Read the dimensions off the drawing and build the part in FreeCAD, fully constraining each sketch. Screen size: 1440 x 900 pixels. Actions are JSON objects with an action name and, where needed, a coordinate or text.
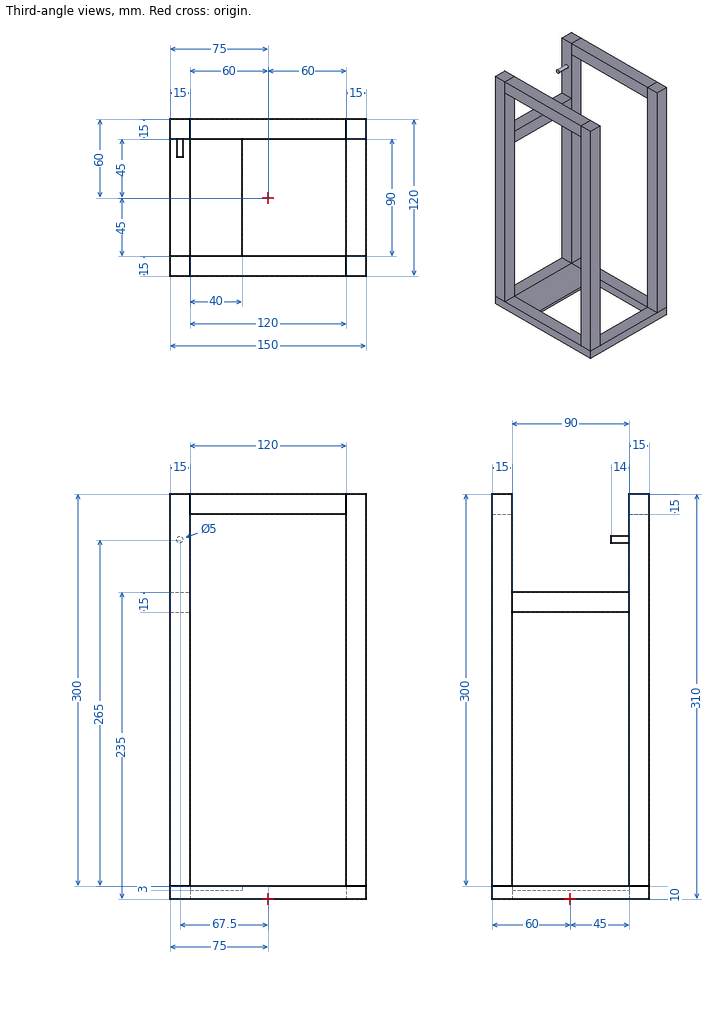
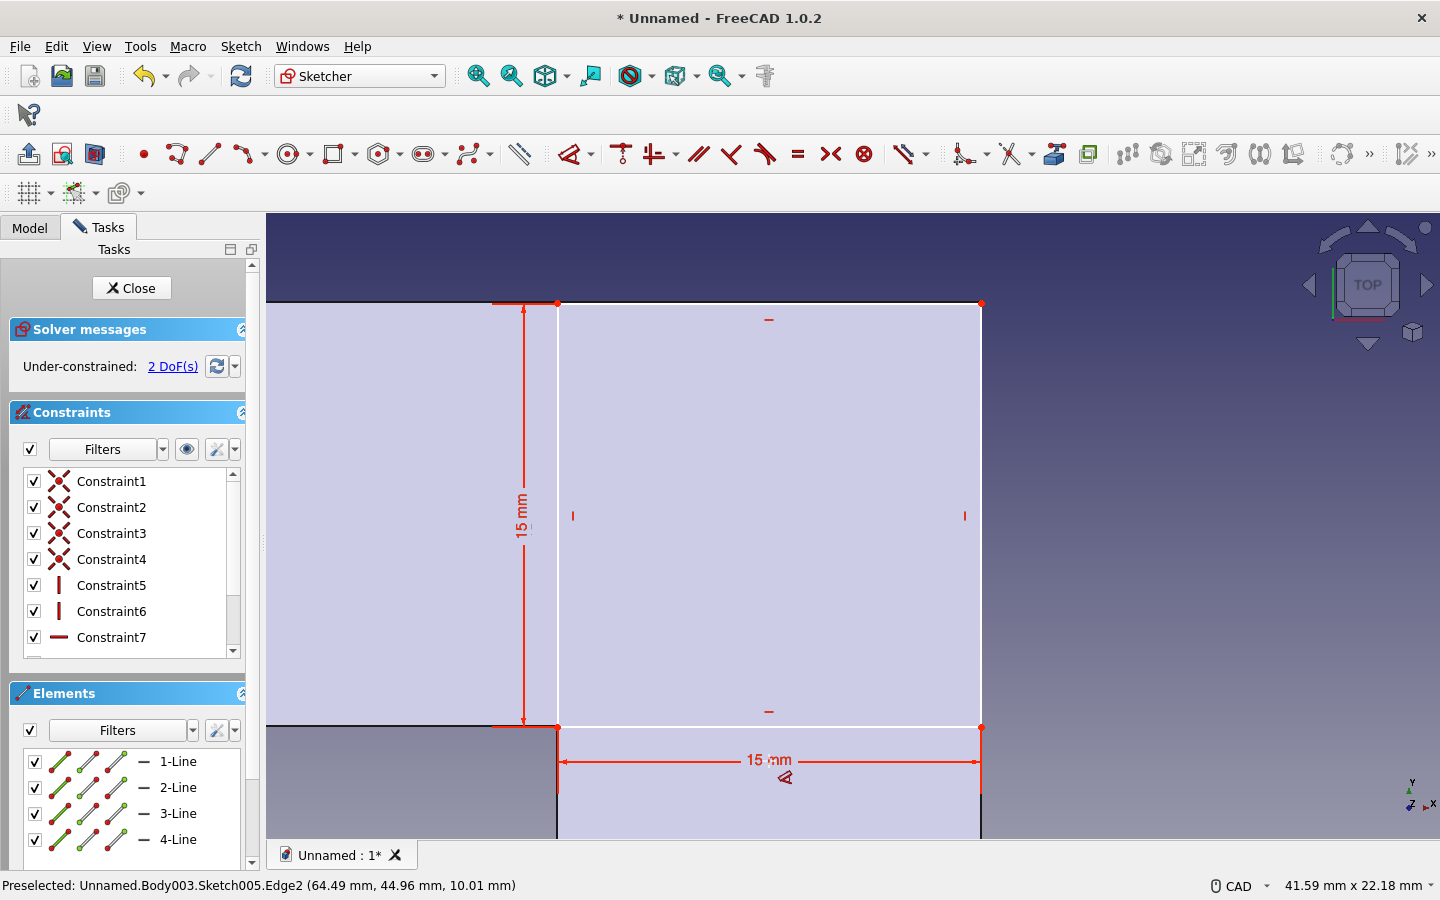
{"action": "left_click", "coordinate": [558, 304]}
{"action": "left_click", "coordinate": [426, 270]}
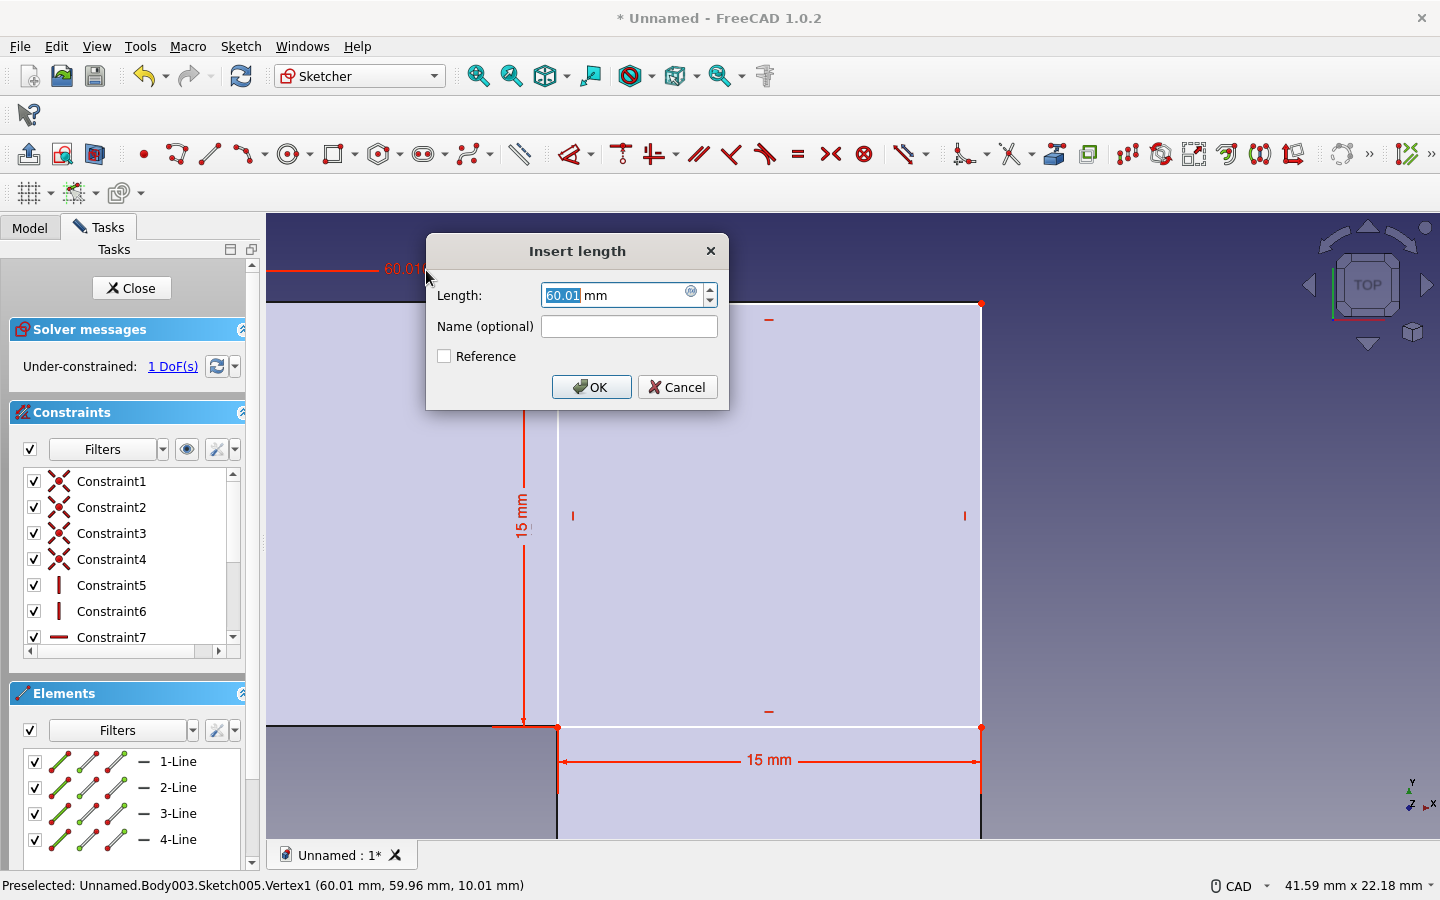
{"action": "type", "text": "60"}
{"action": "key", "text": "Return"}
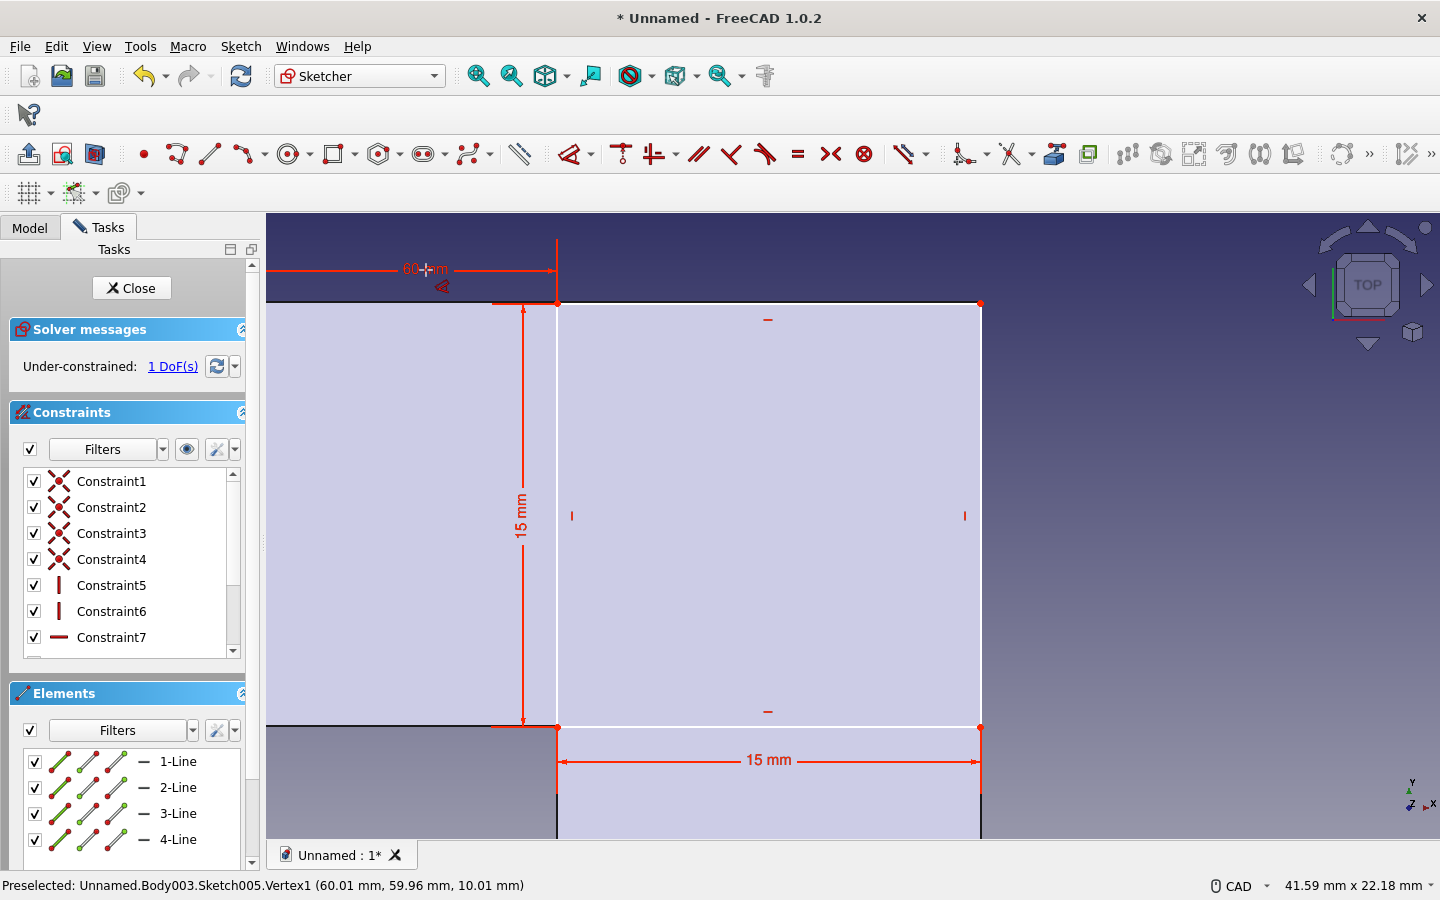
{"action": "left_click", "coordinate": [557, 304]}
{"action": "left_click", "coordinate": [591, 557]}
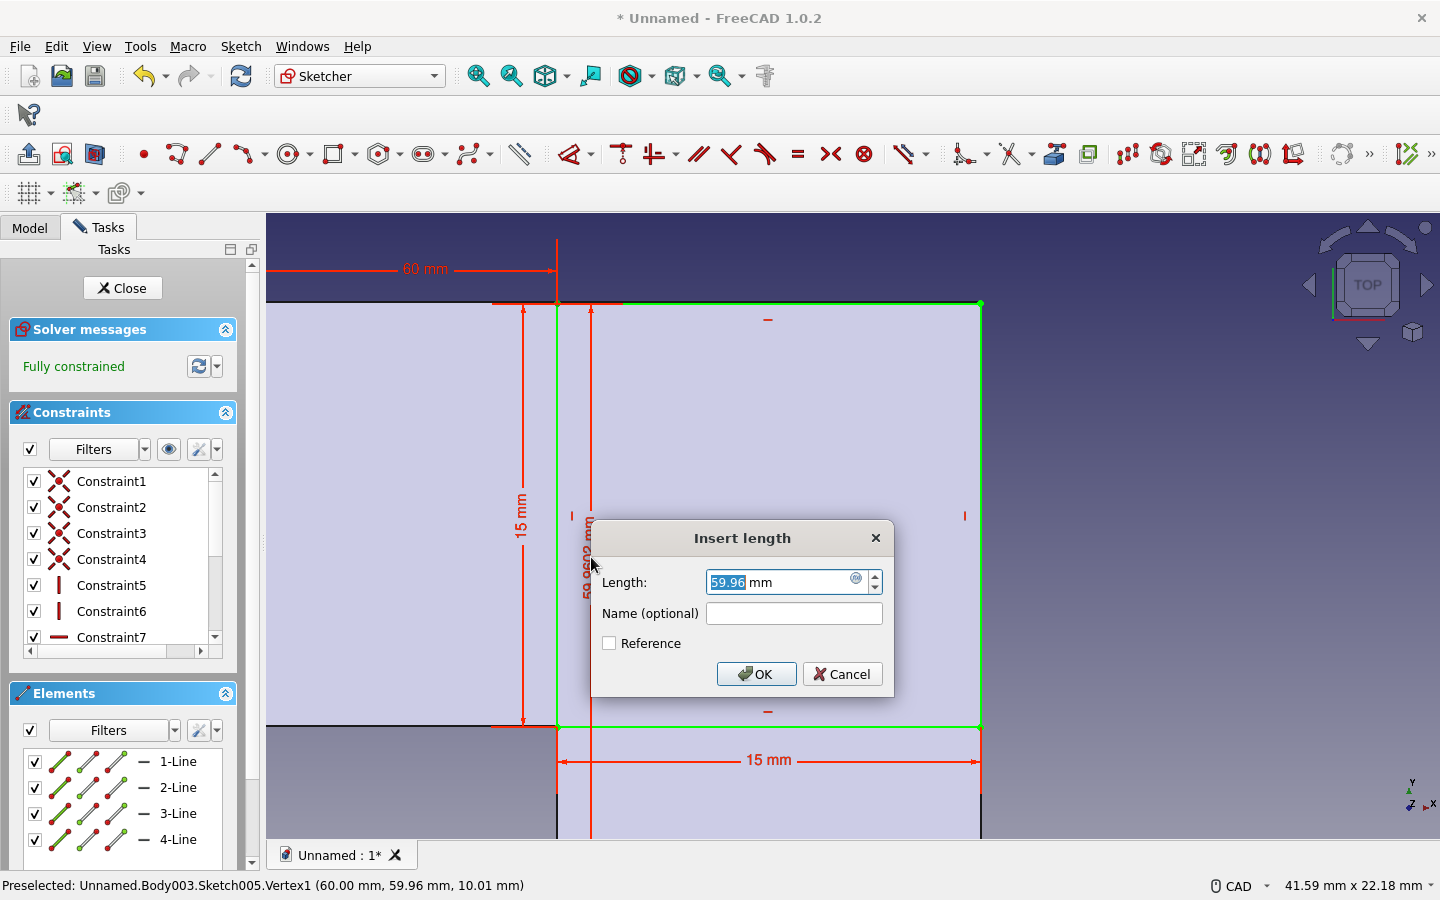
{"action": "type", "text": "60"}
{"action": "key", "text": "Return"}
{"action": "key", "text": "Escape"}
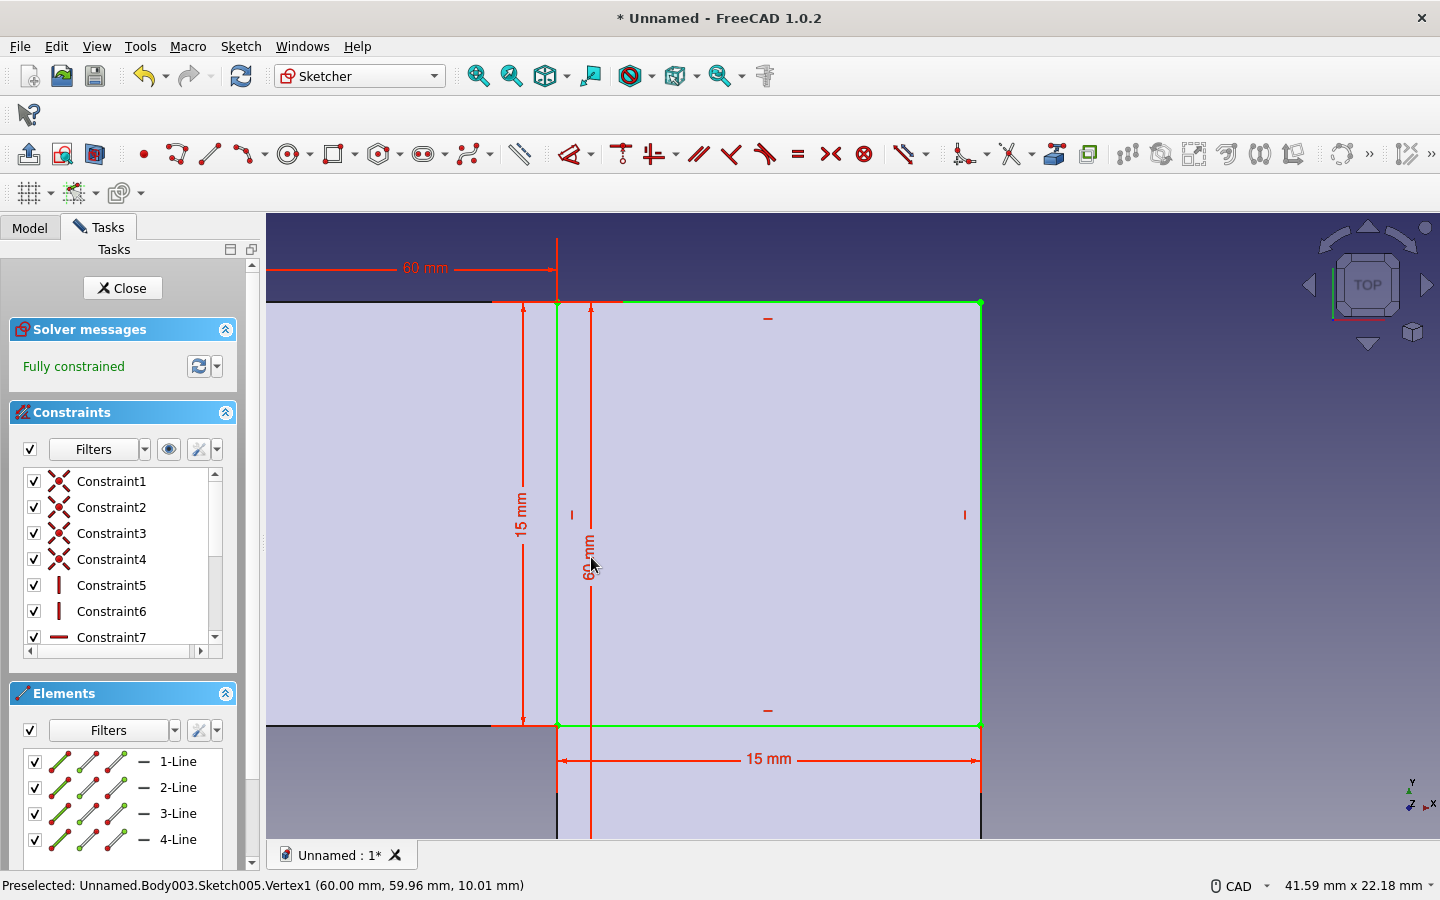
{"action": "left_click", "coordinate": [123, 288]}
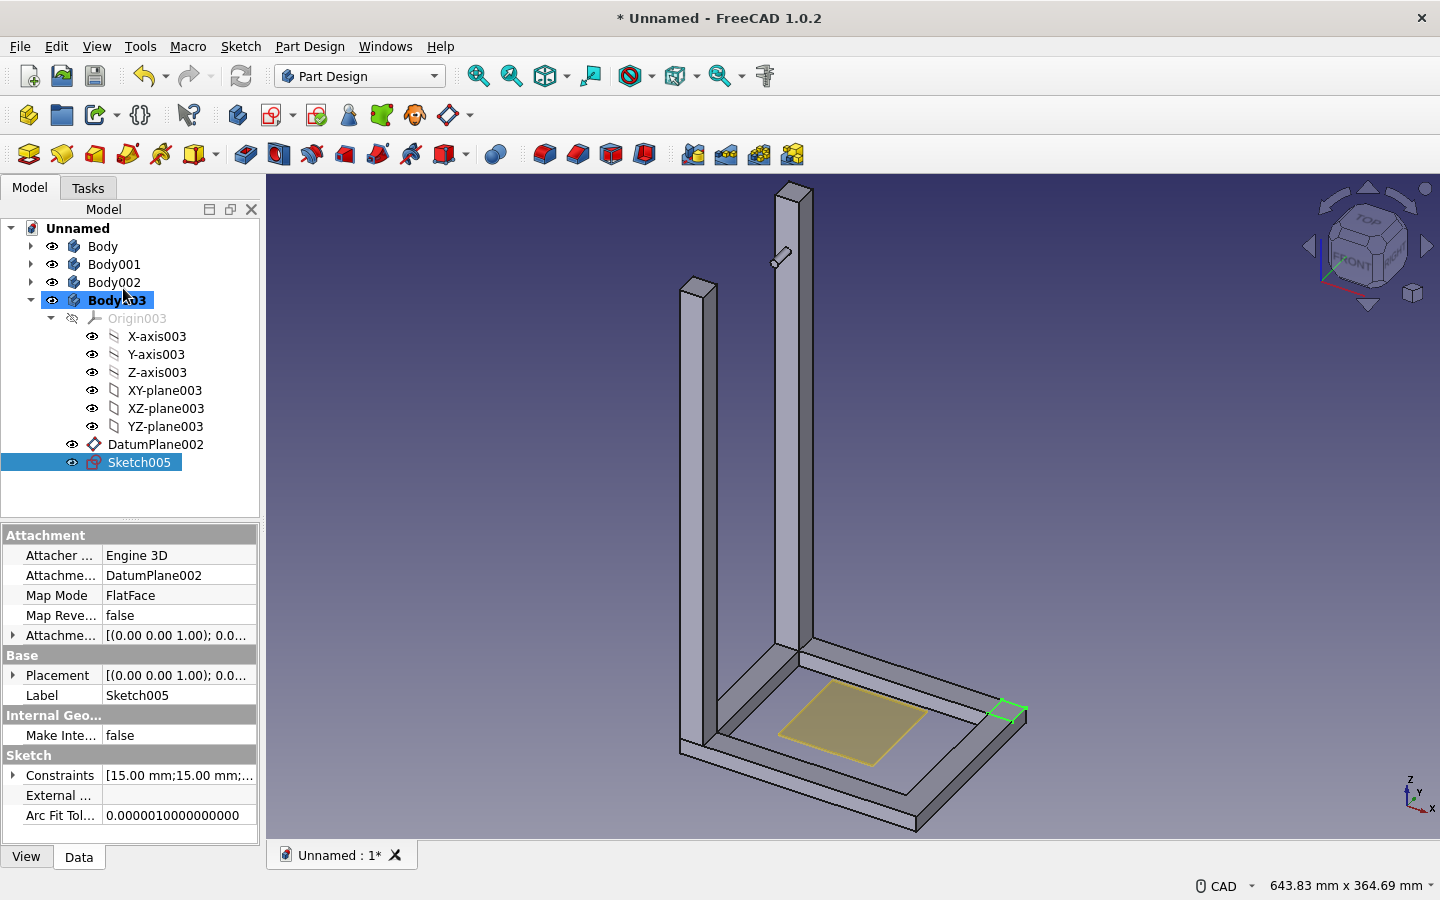
{"action": "left_click", "coordinate": [29, 154]}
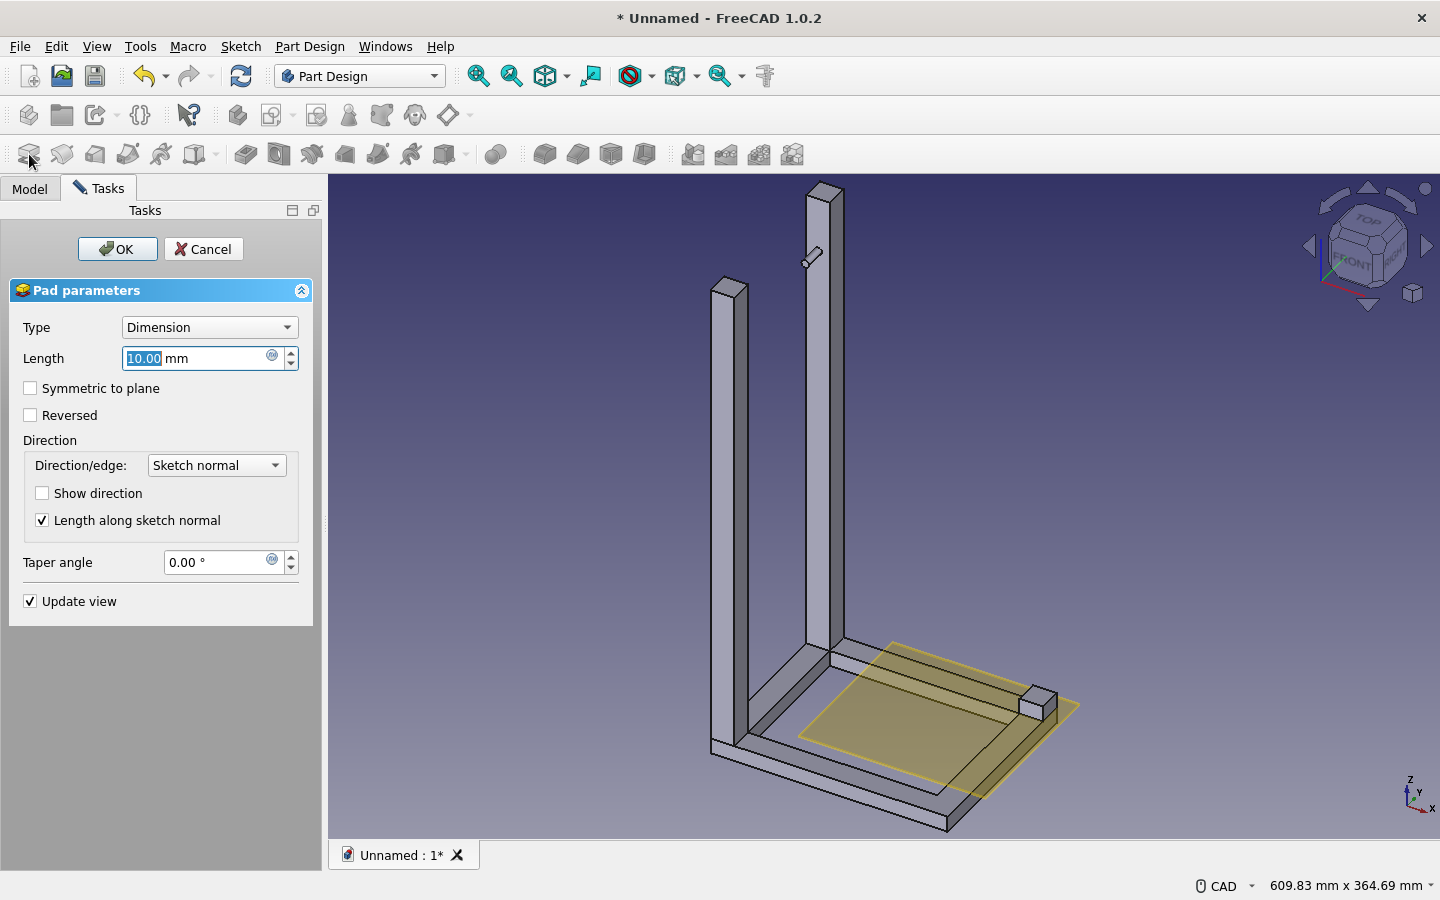
{"action": "type", "text": "300"}
{"action": "key", "text": "Tab"}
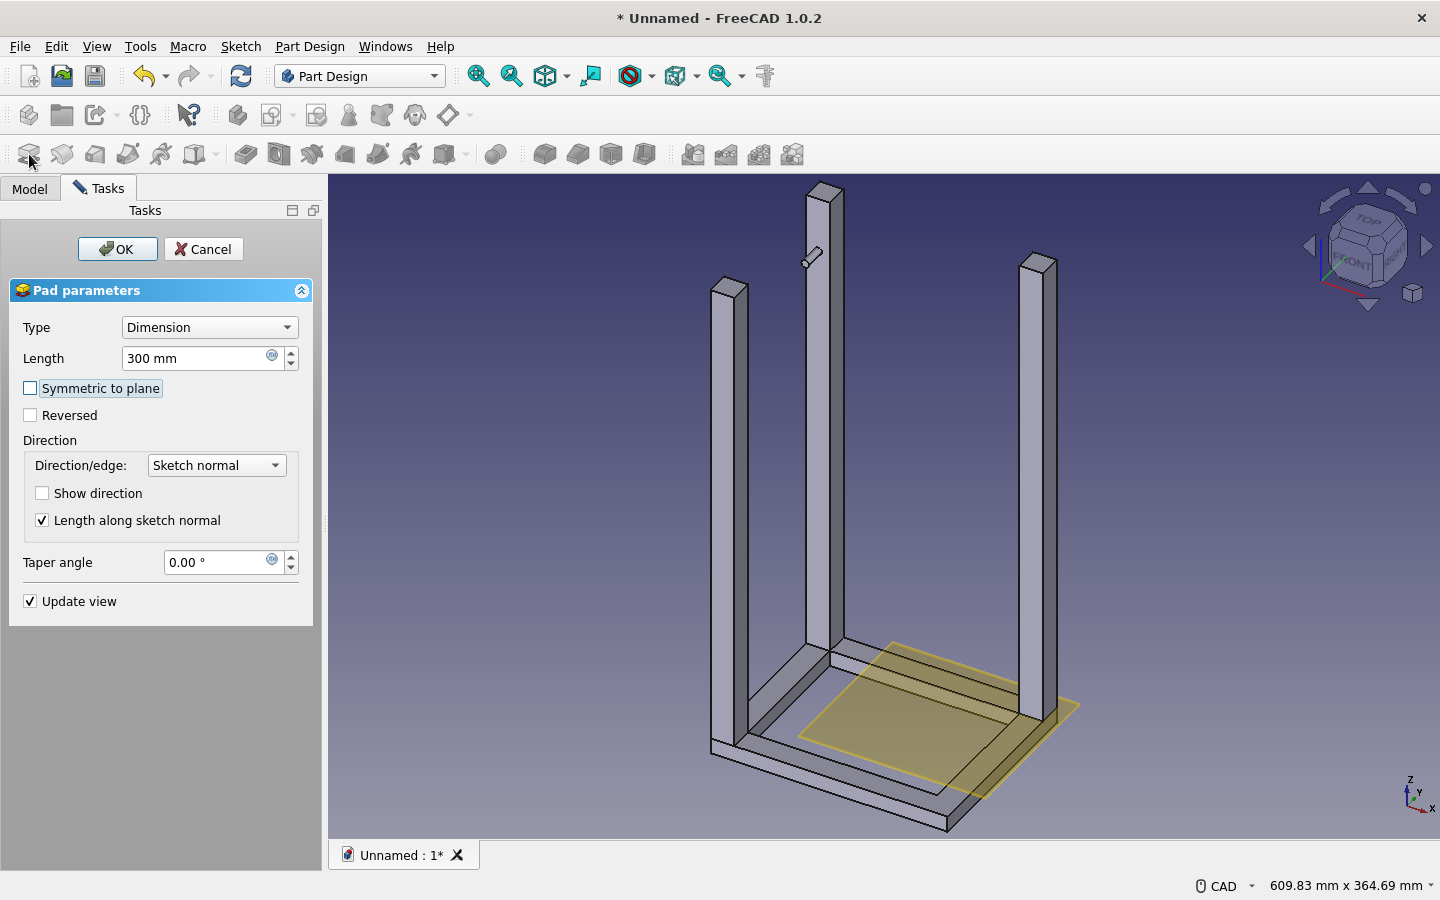
{"action": "left_click", "coordinate": [118, 249]}